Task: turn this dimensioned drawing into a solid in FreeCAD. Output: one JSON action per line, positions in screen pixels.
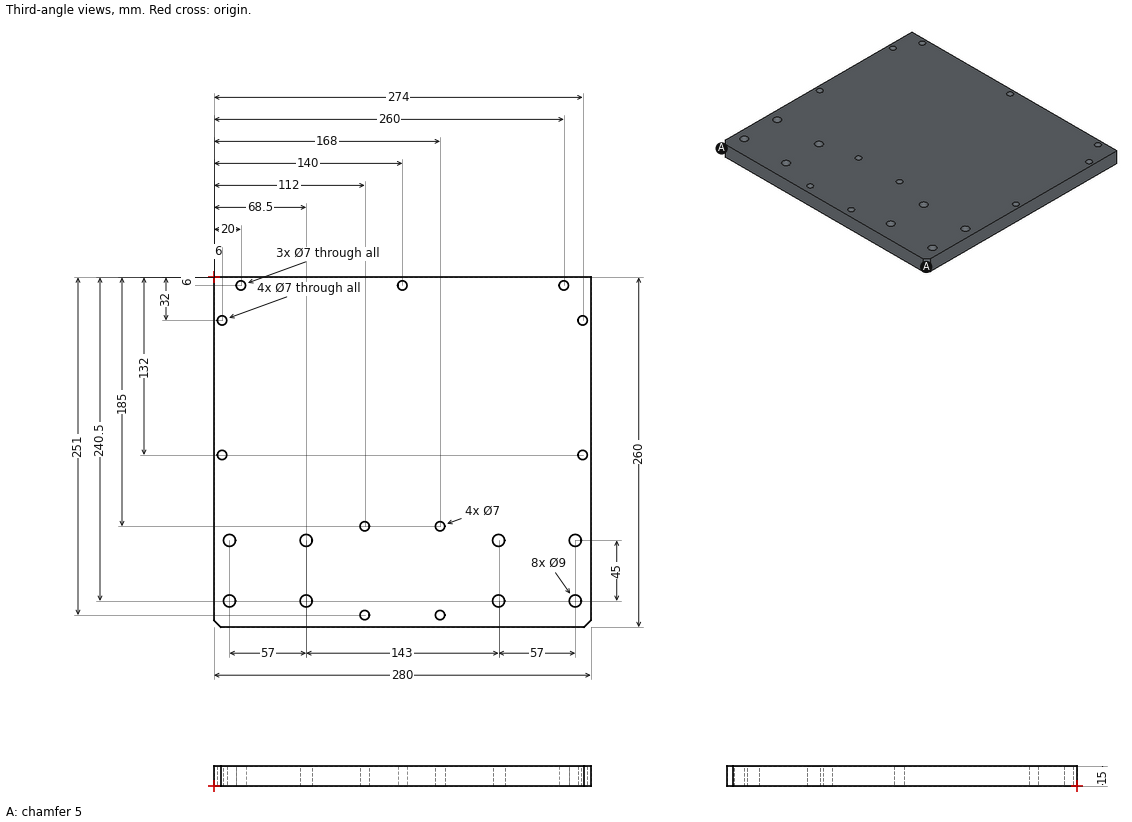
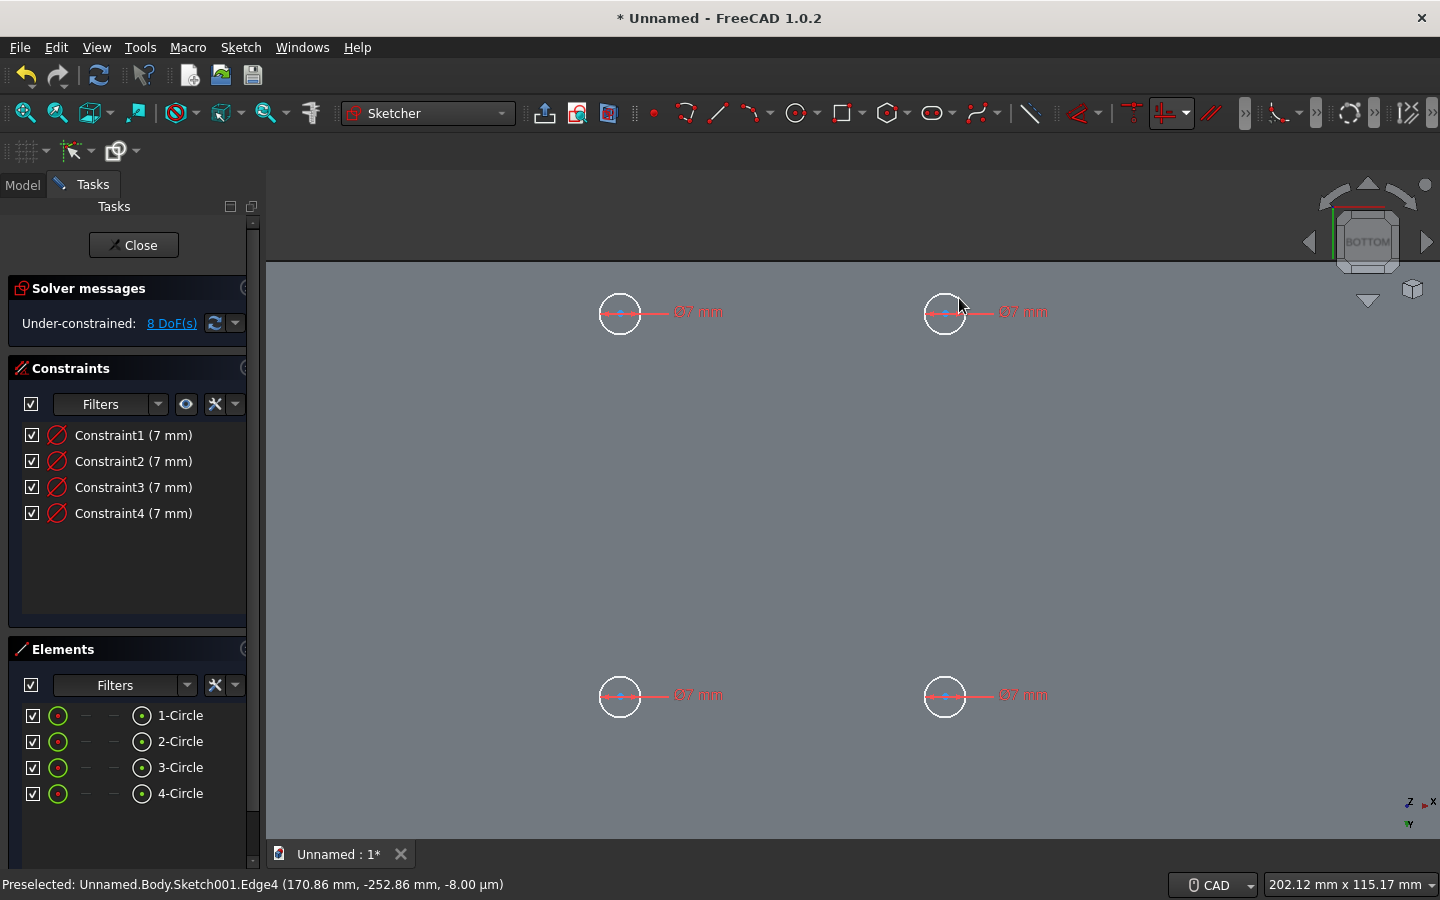
{"action": "left_click", "coordinate": [945, 697]}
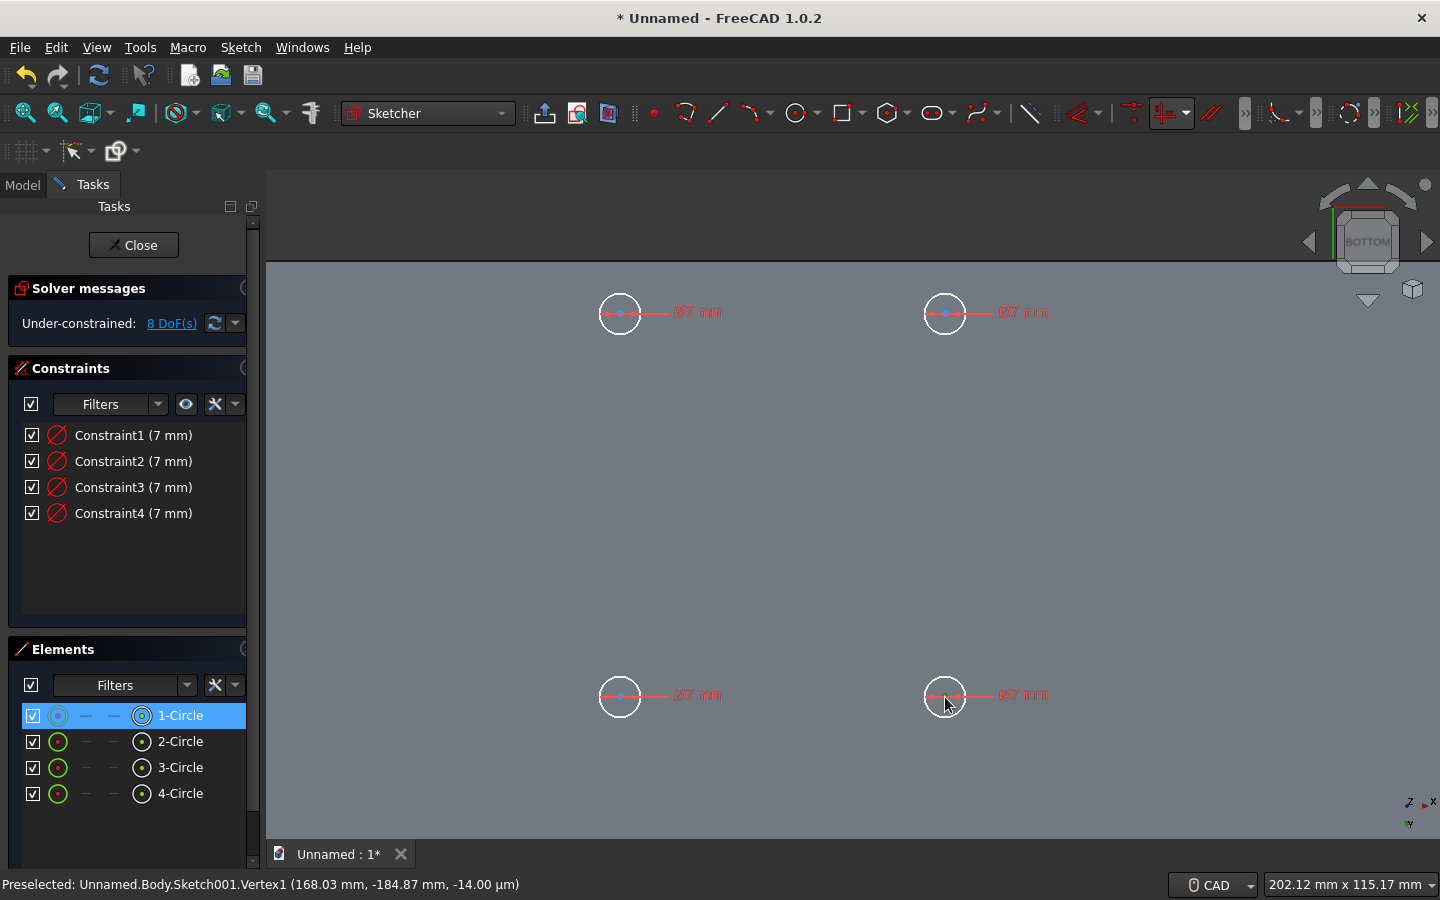
{"action": "left_click", "coordinate": [620, 697]}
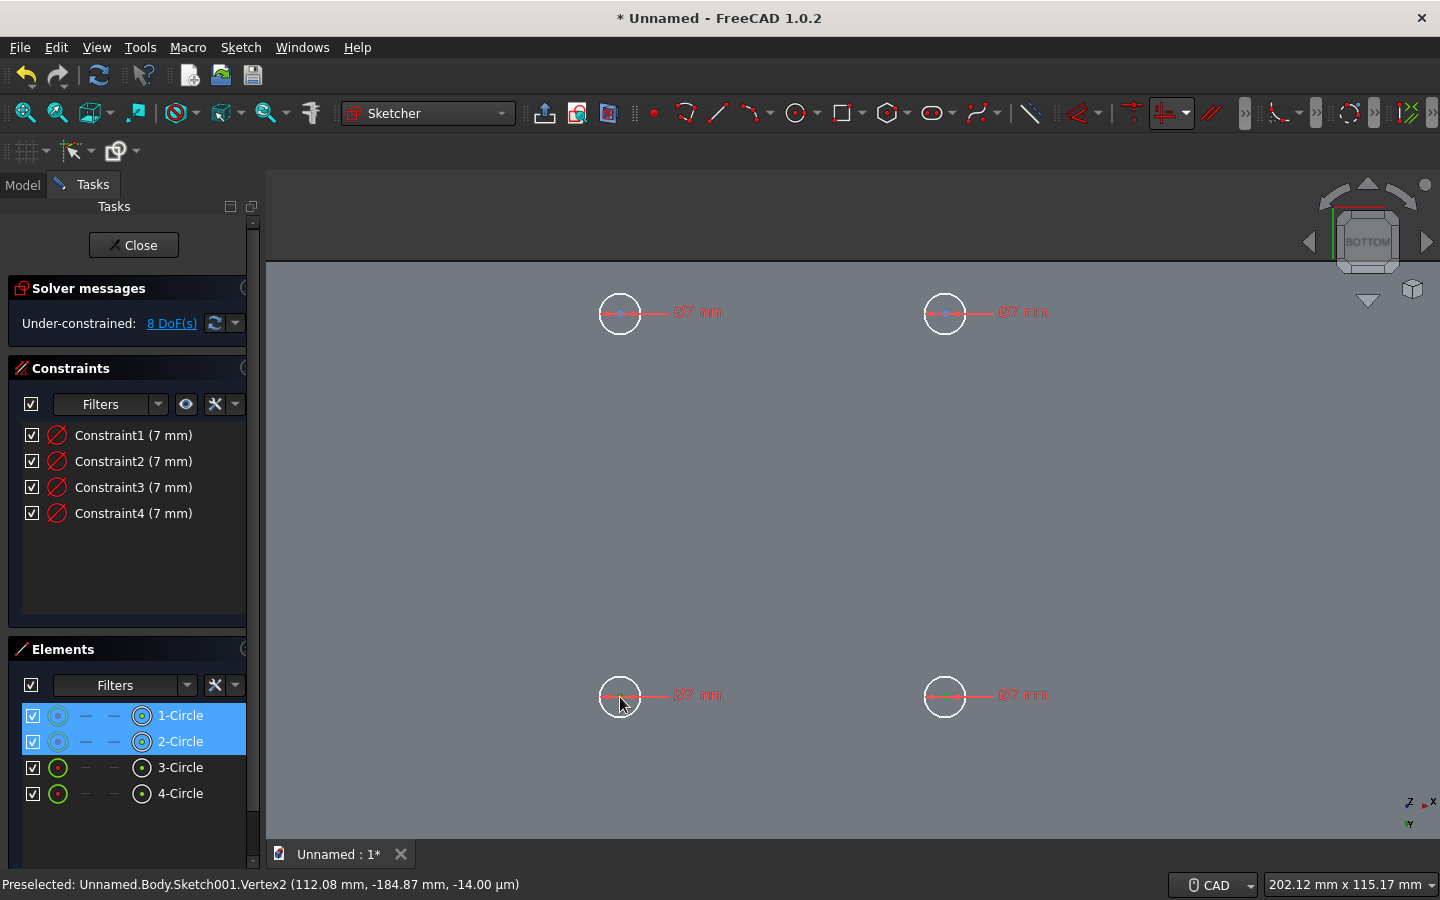
{"action": "left_click", "coordinate": [1188, 114]}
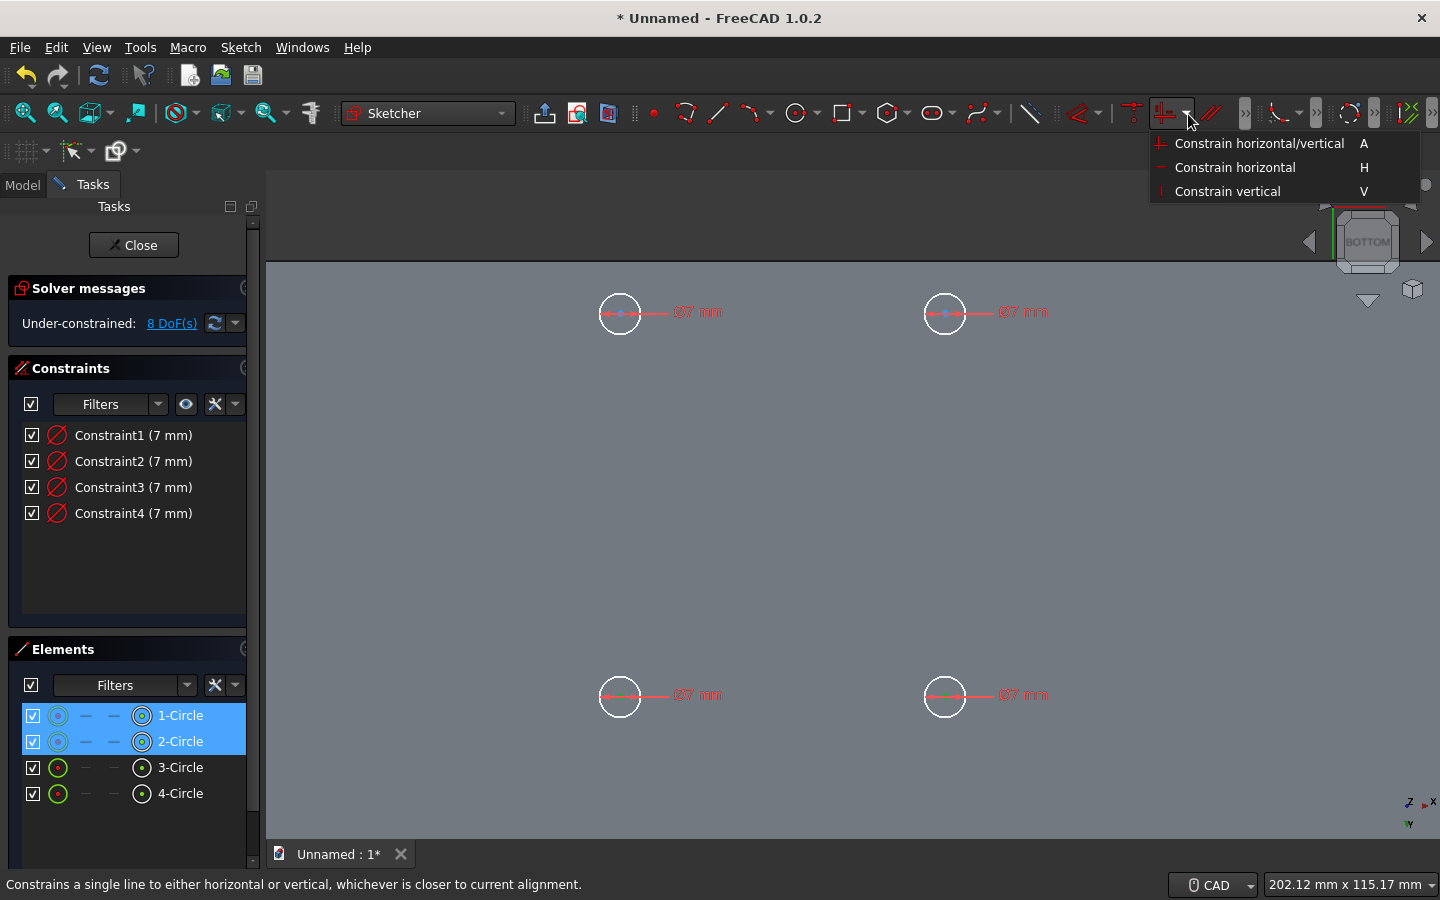
{"action": "left_click", "coordinate": [1285, 167]}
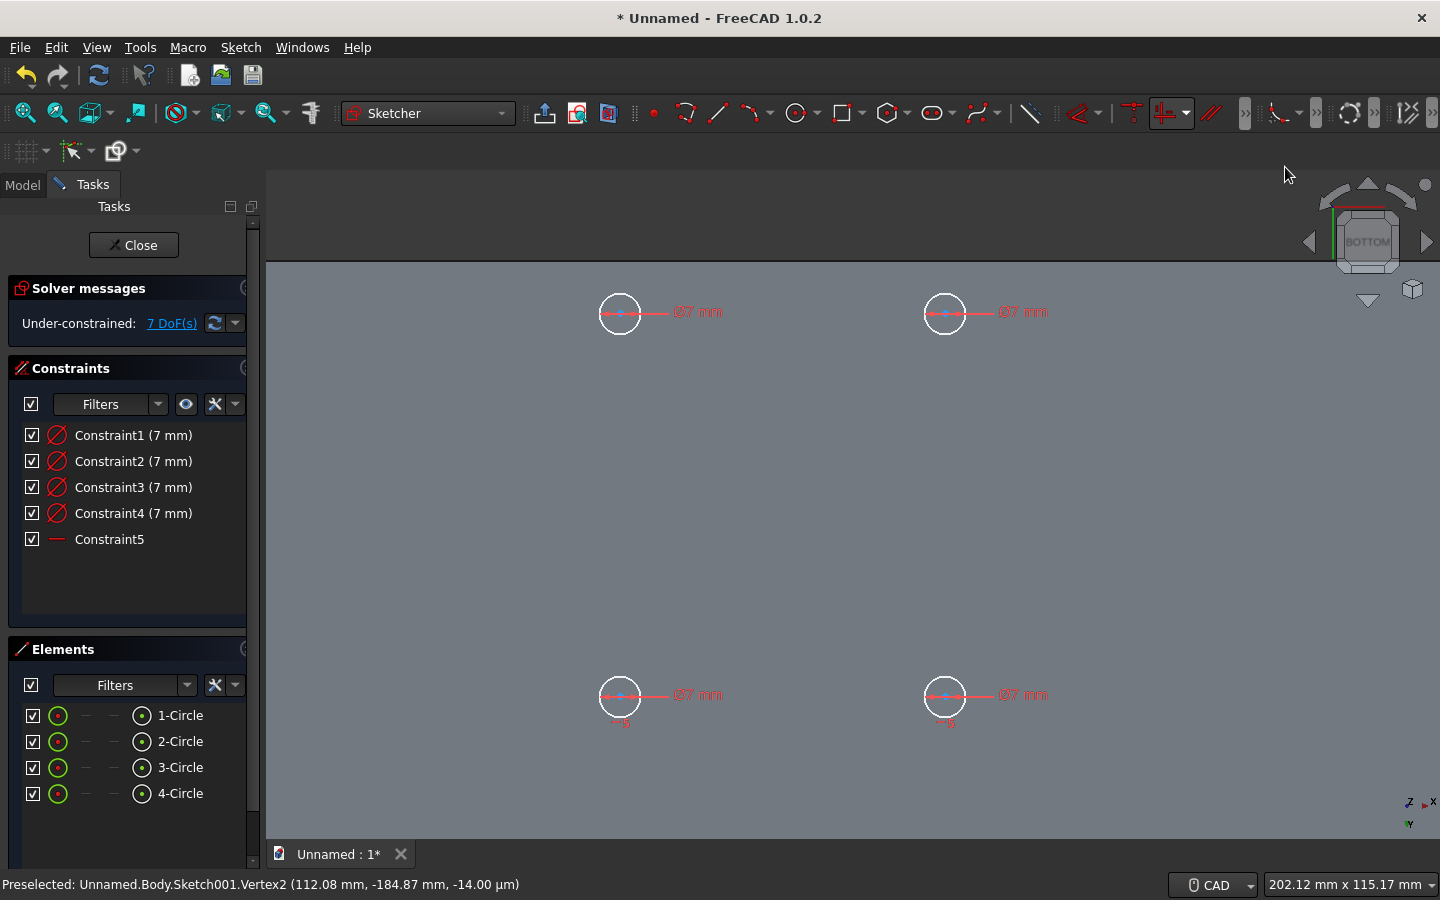
{"action": "left_click", "coordinate": [620, 697]}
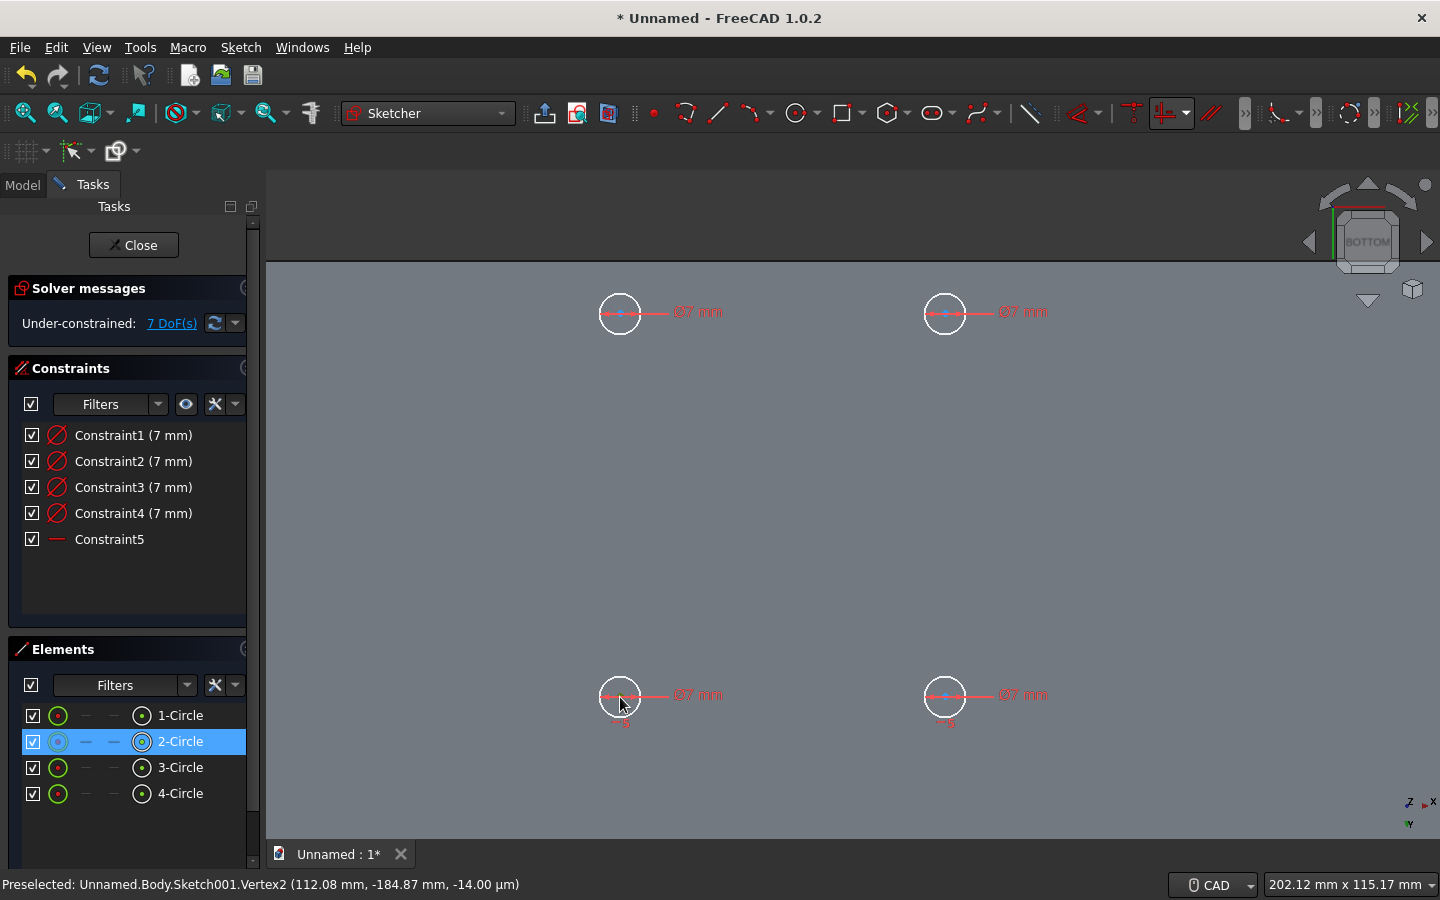
{"action": "left_click", "coordinate": [620, 314]}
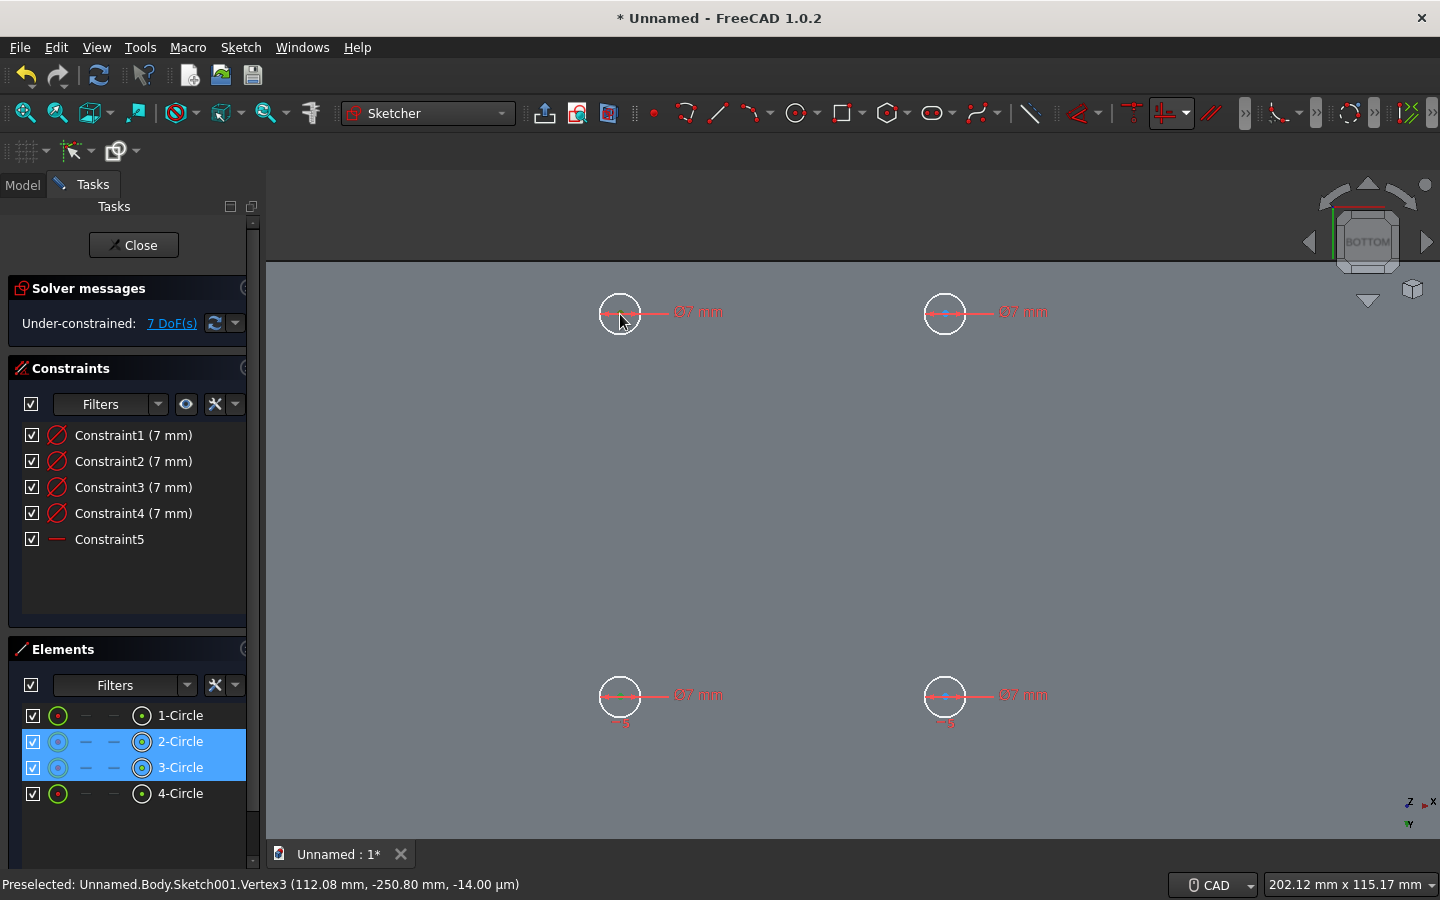
{"action": "key", "text": "v"}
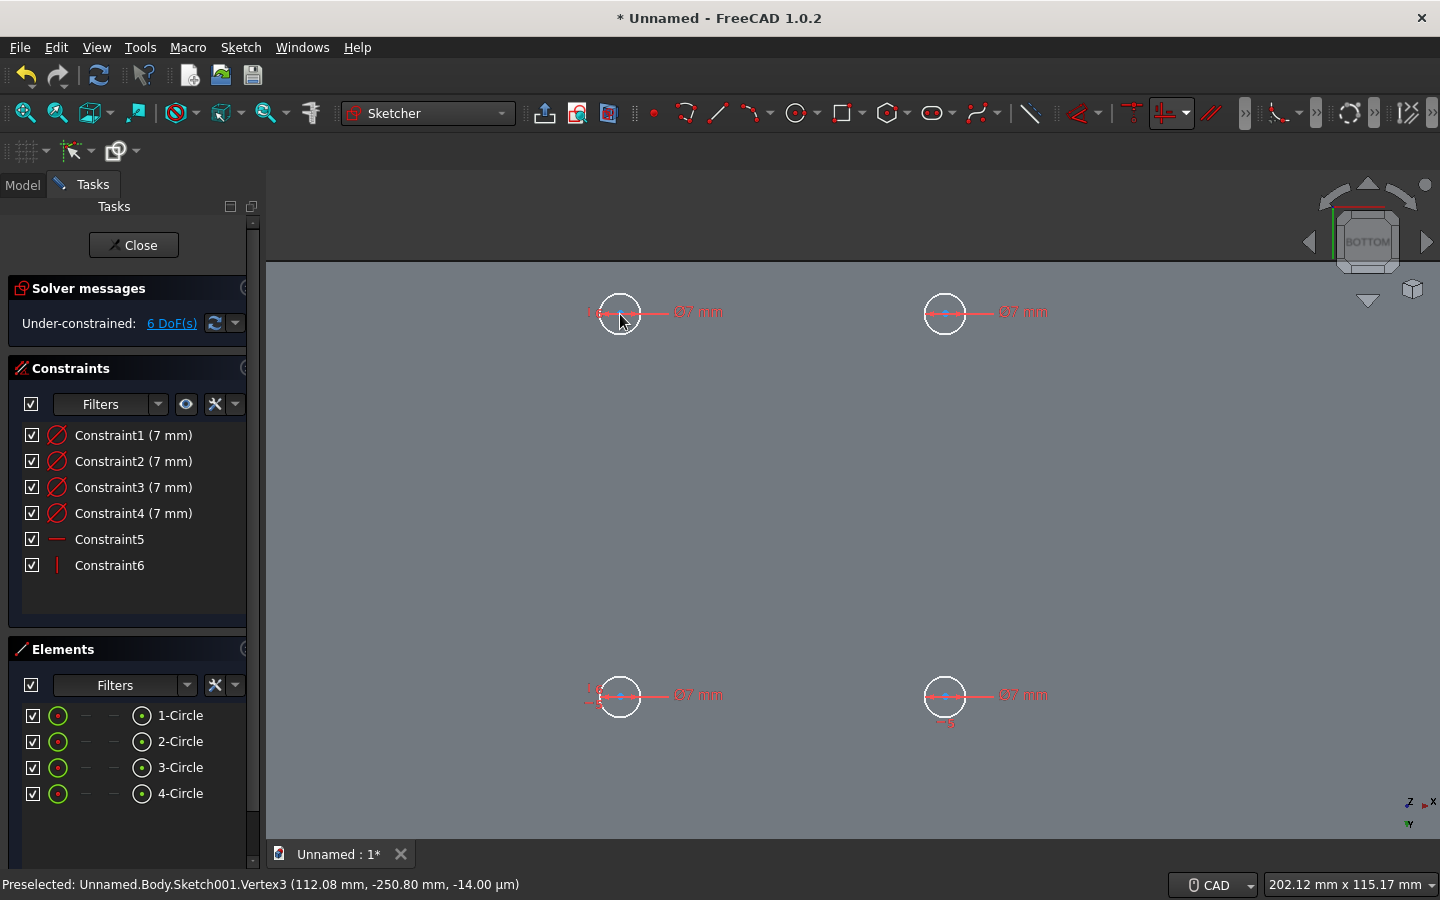
{"action": "left_click", "coordinate": [945, 697]}